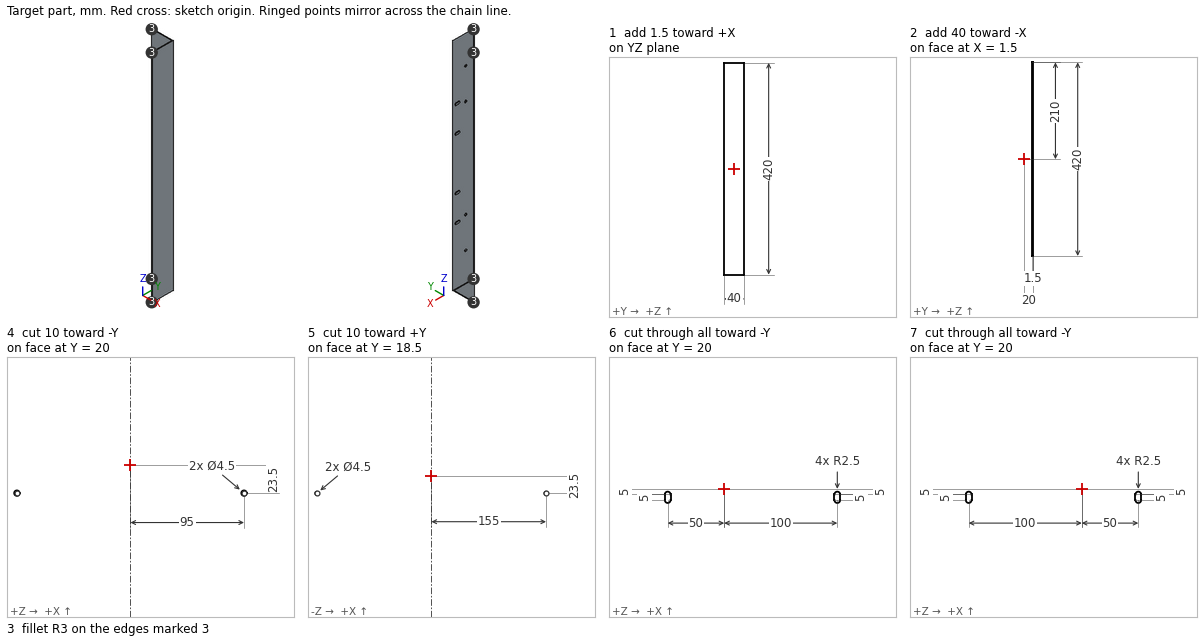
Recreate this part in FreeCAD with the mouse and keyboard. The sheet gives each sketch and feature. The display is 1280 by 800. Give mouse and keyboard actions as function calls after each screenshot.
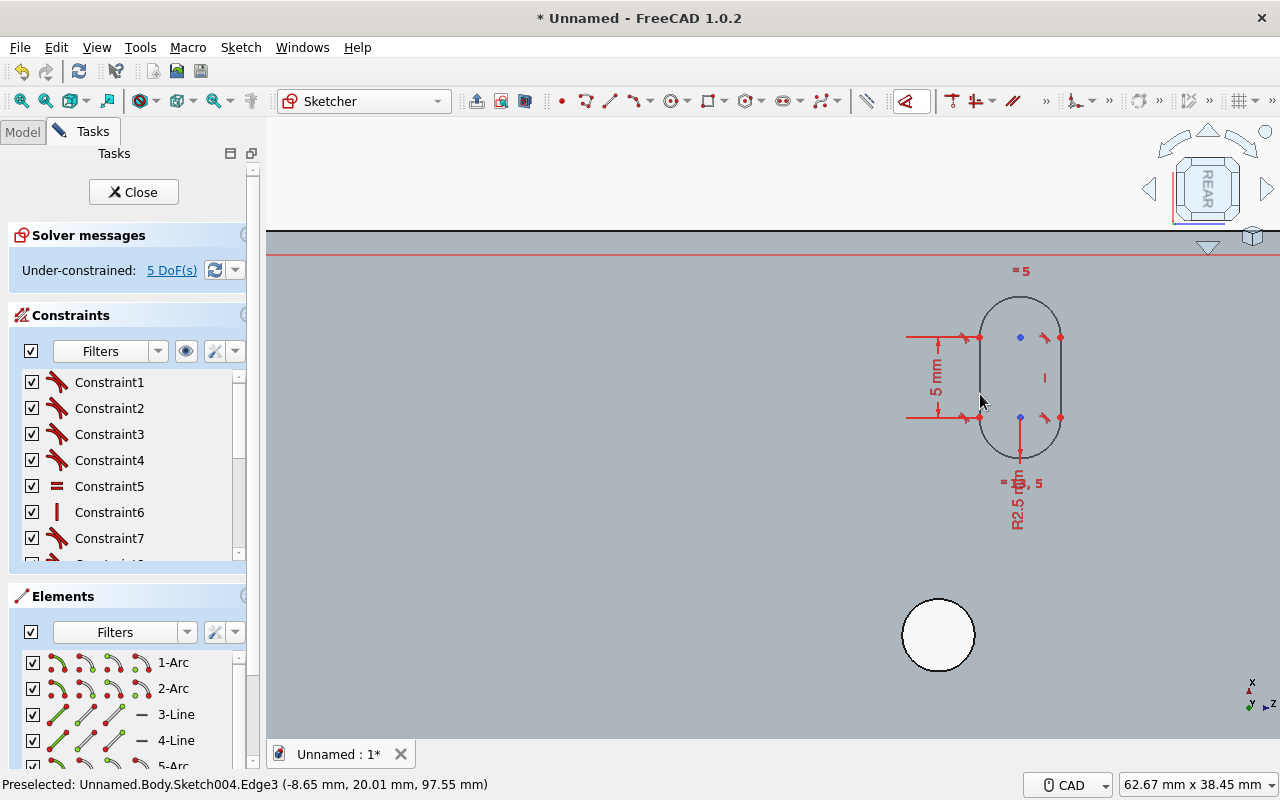
scroll(999, 452, down, 7)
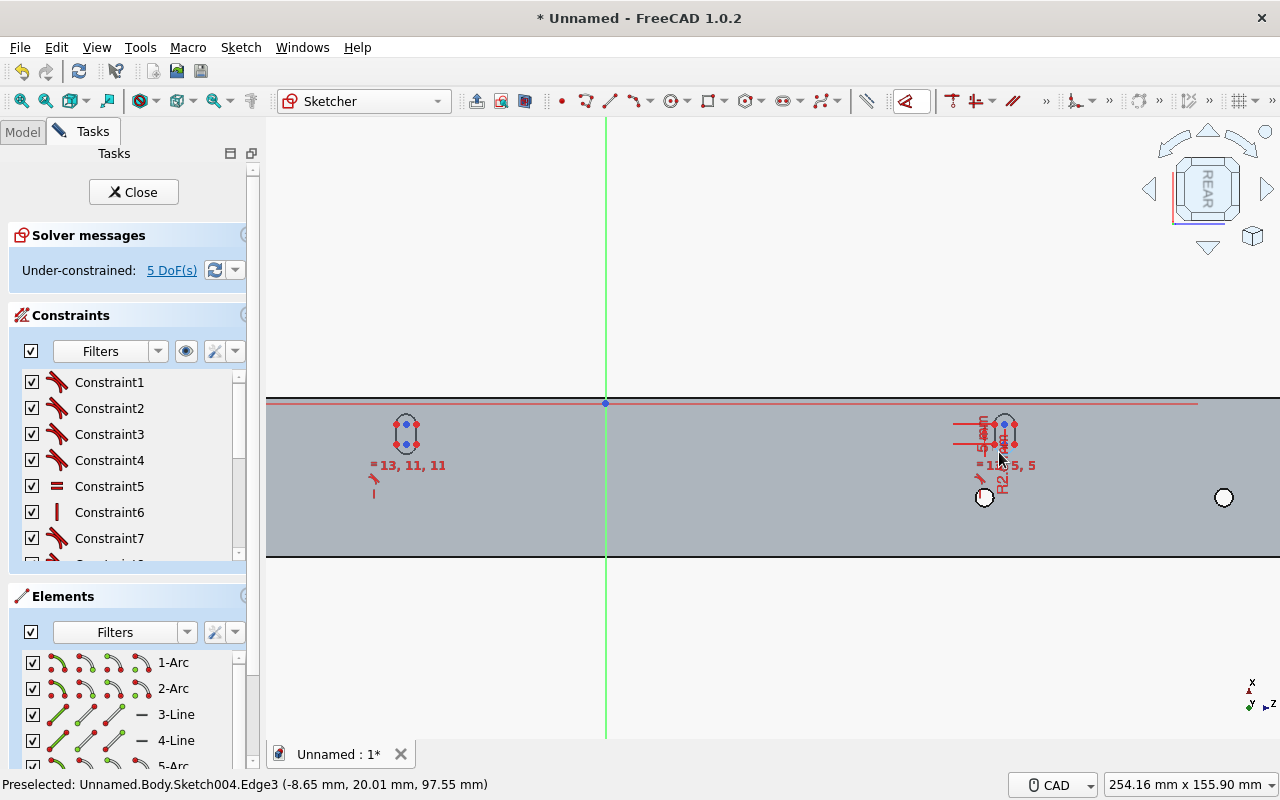
scroll(396, 438, up, 5)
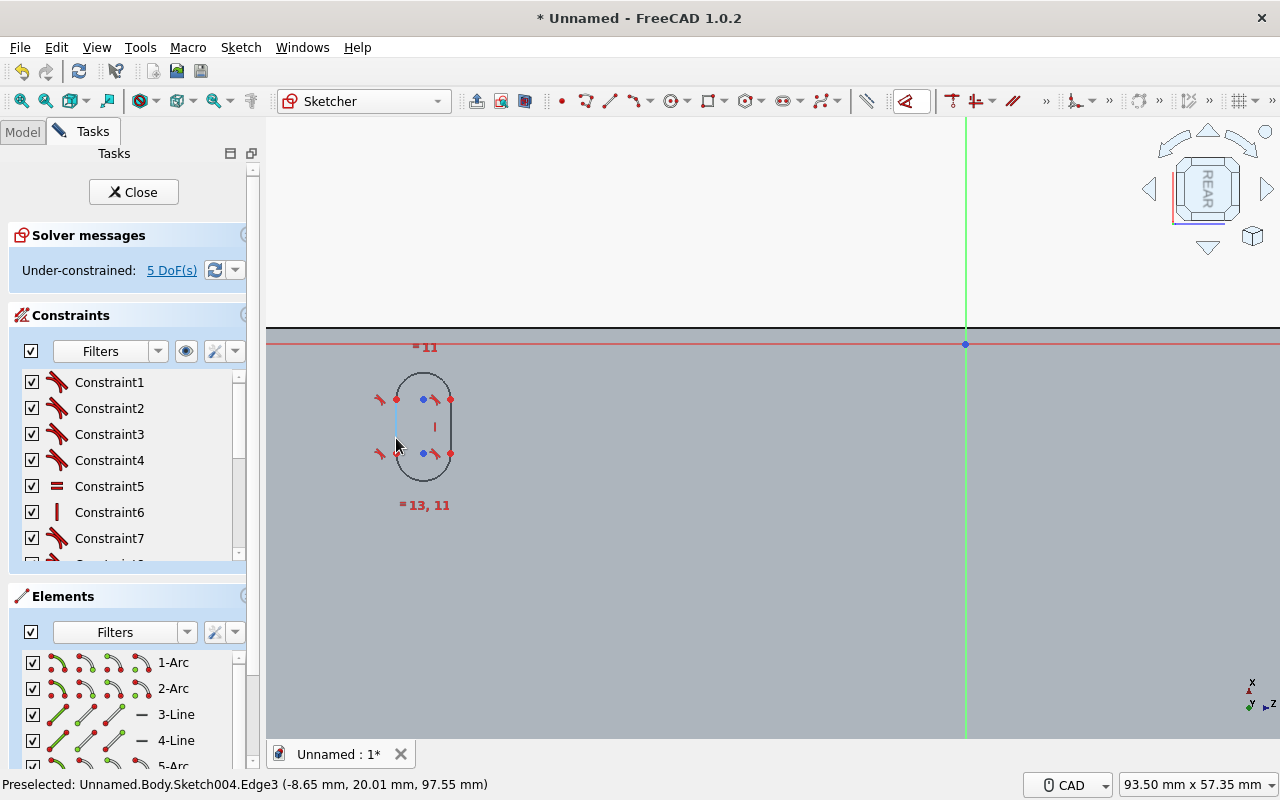
click(396, 438)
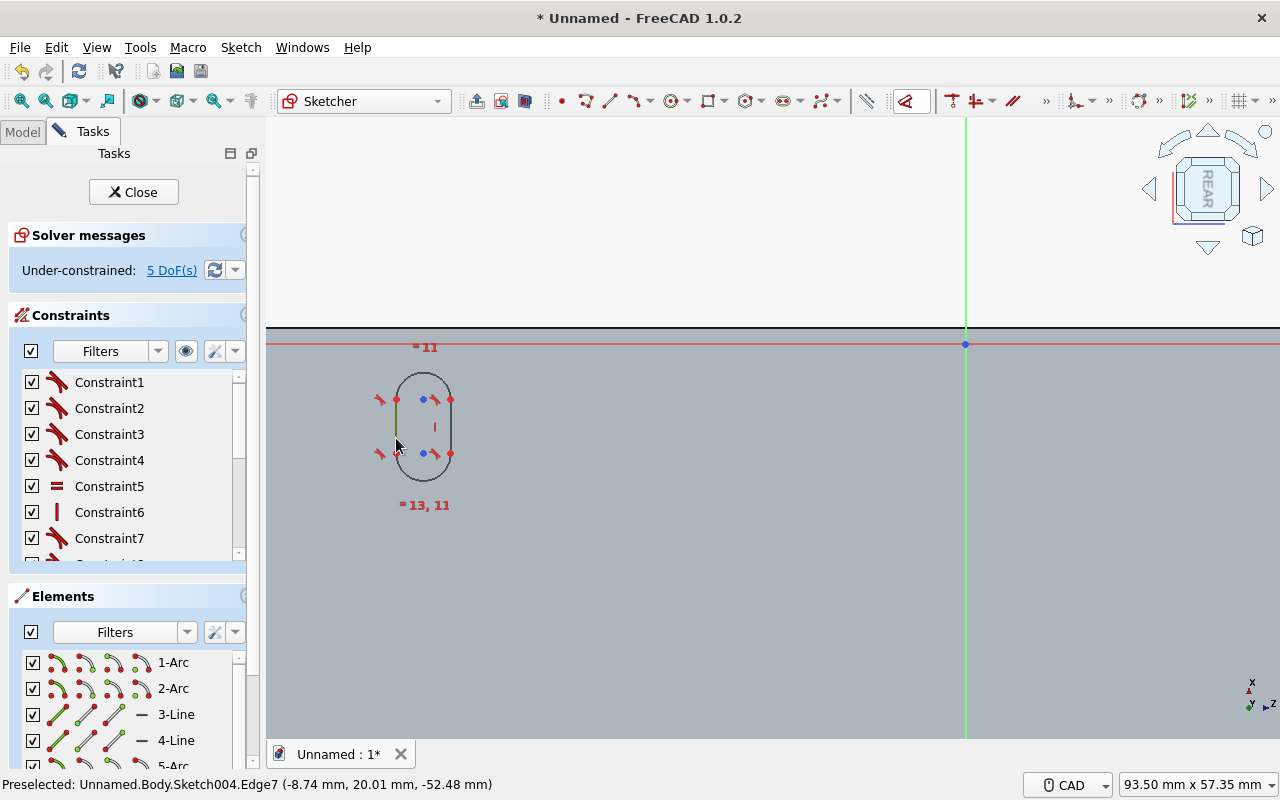
key(i)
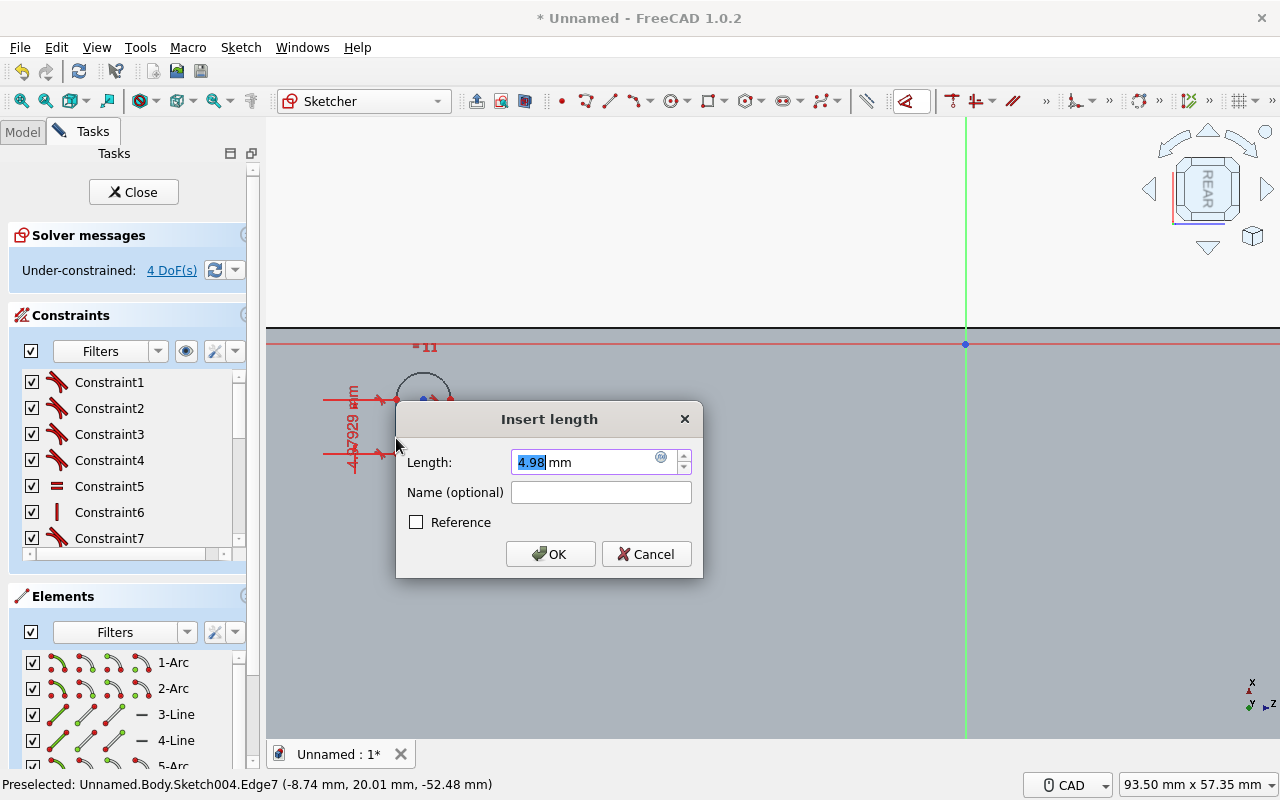
text(5)
key(Return)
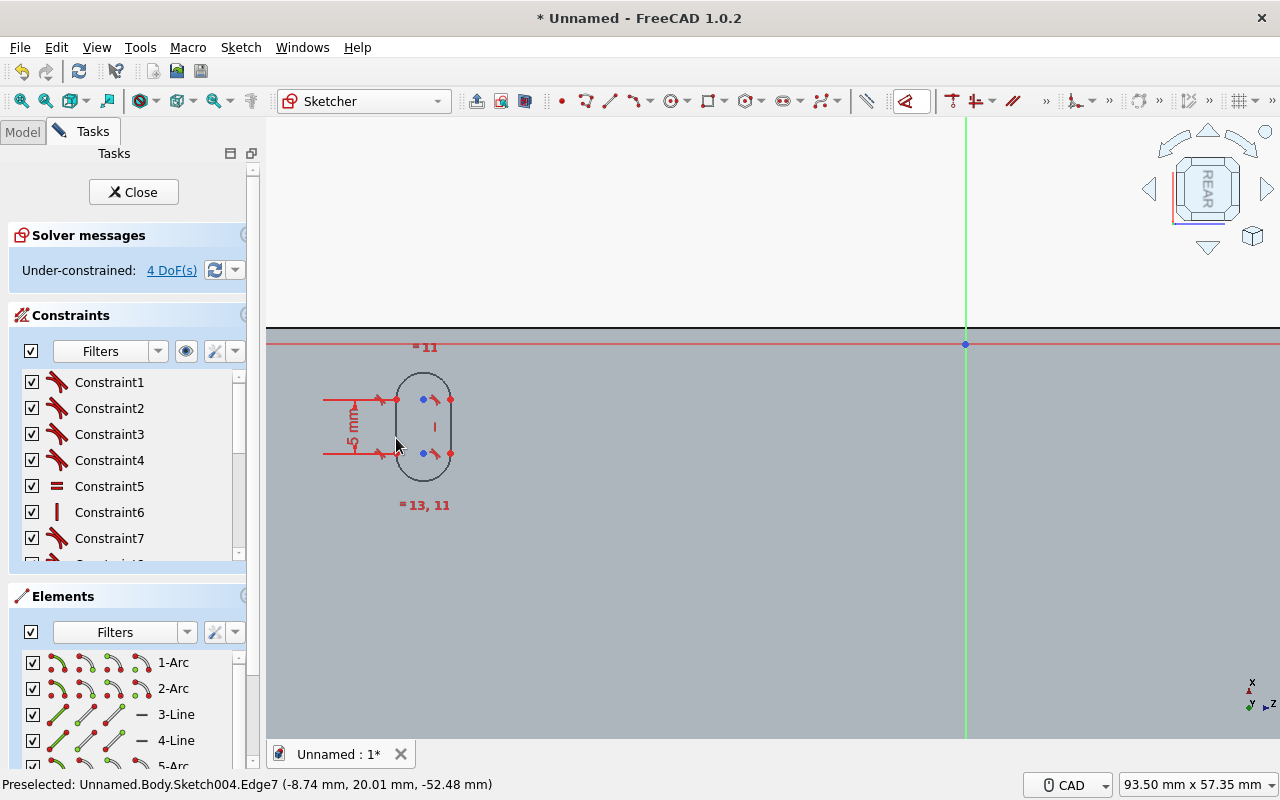
scroll(395, 437, down, 5)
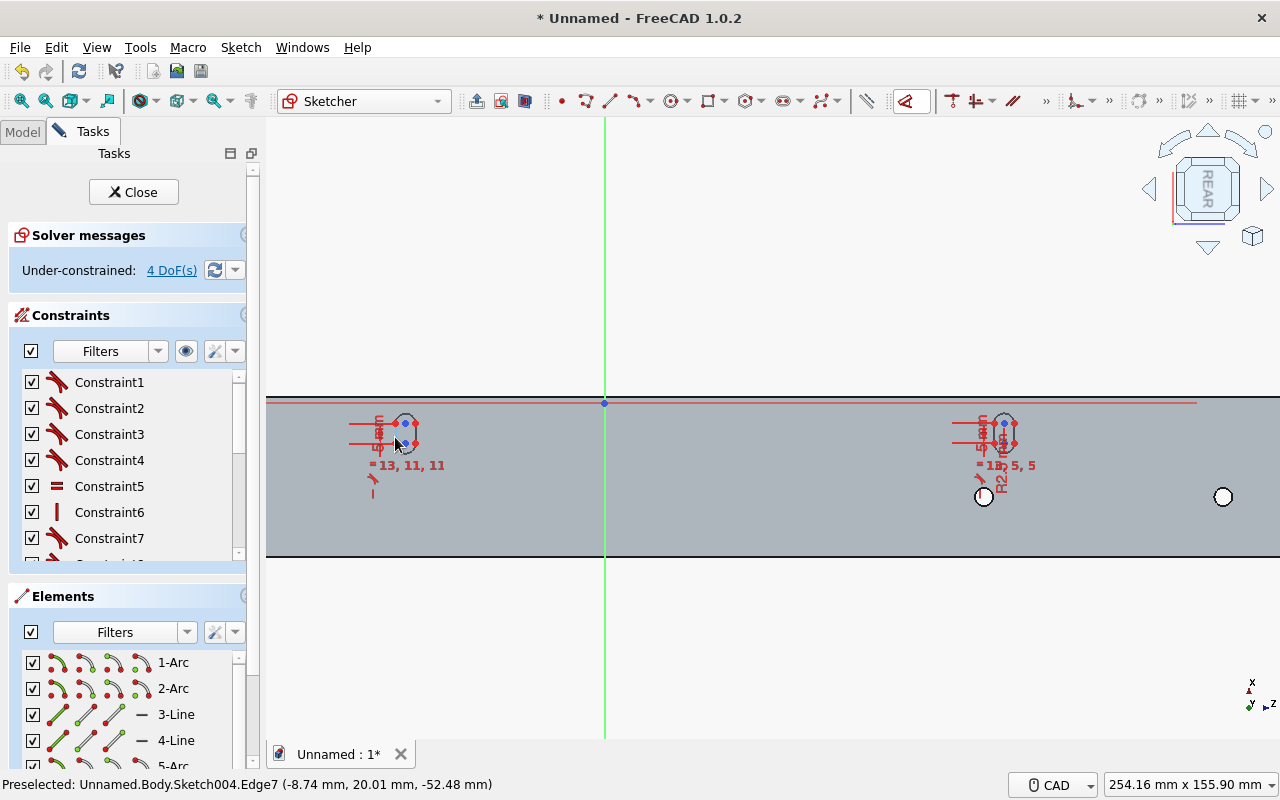
scroll(1014, 423, up, 4)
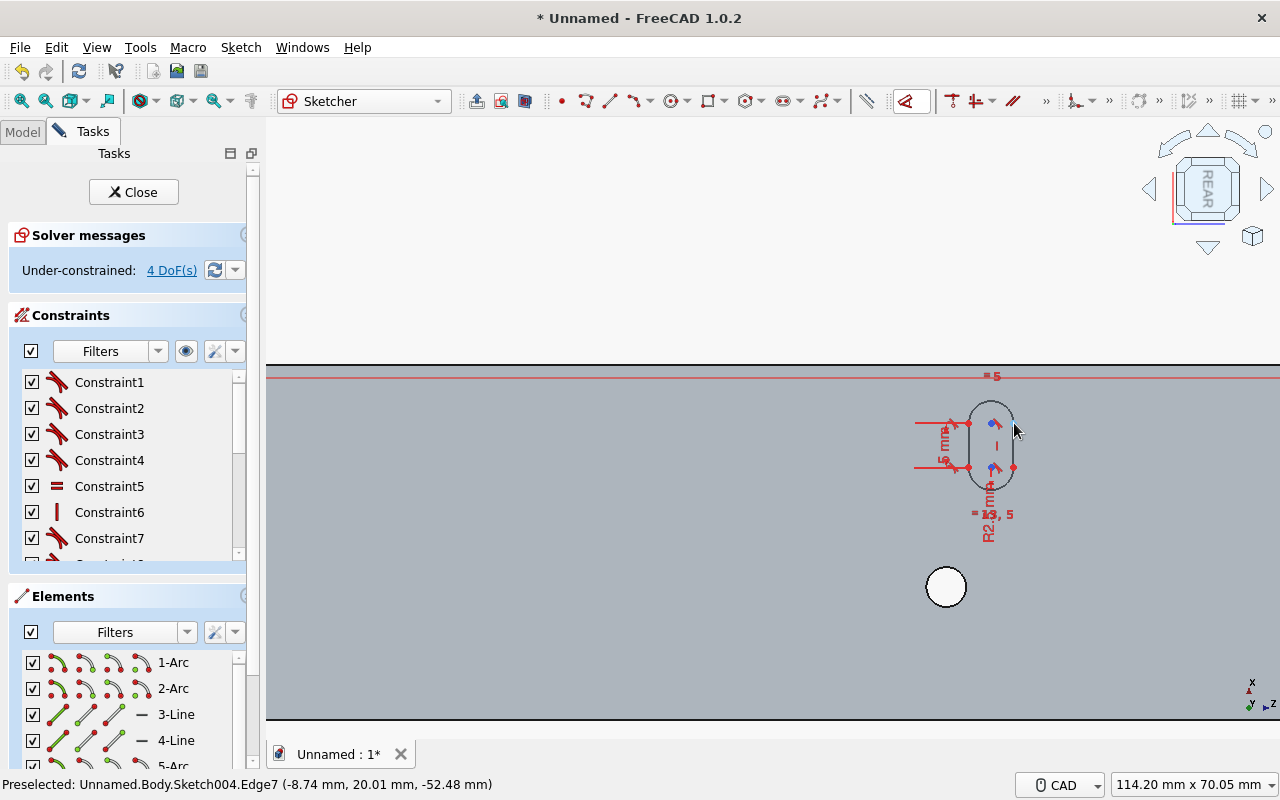
click(1013, 423)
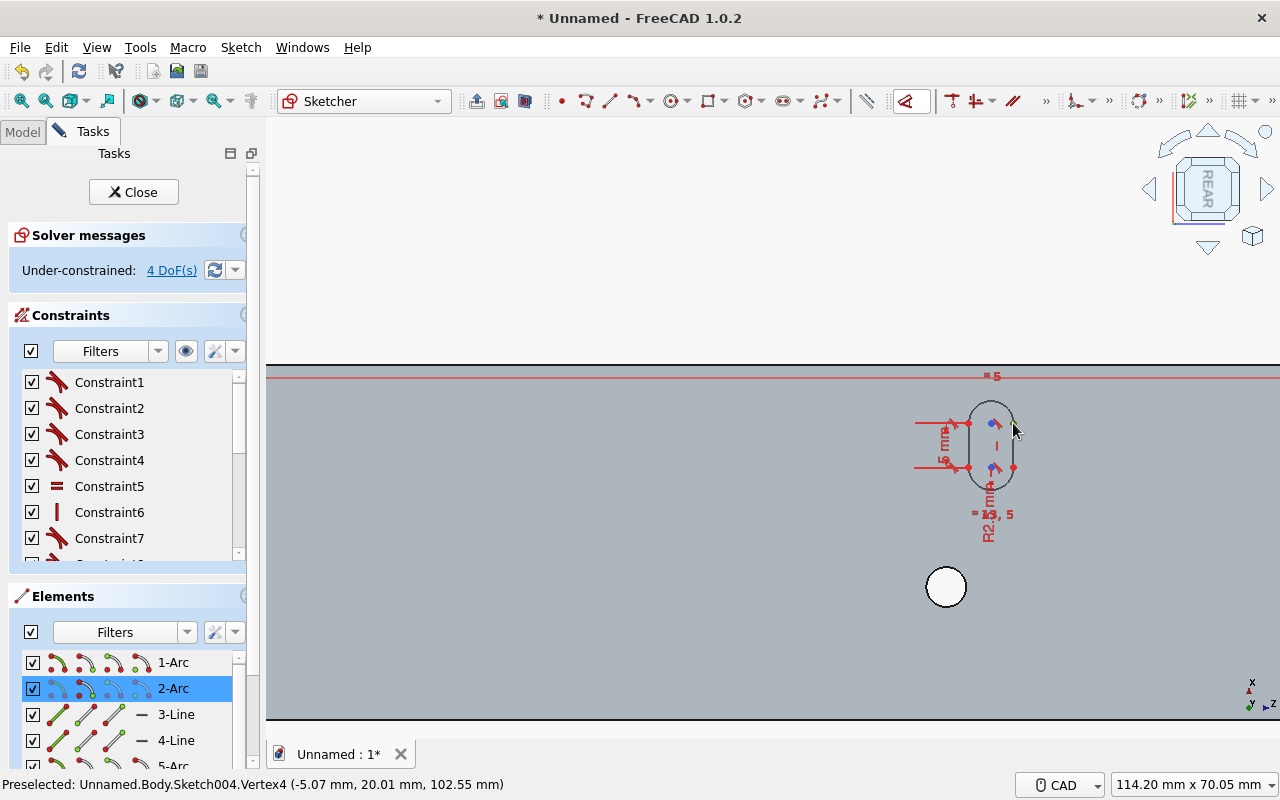
click(924, 102)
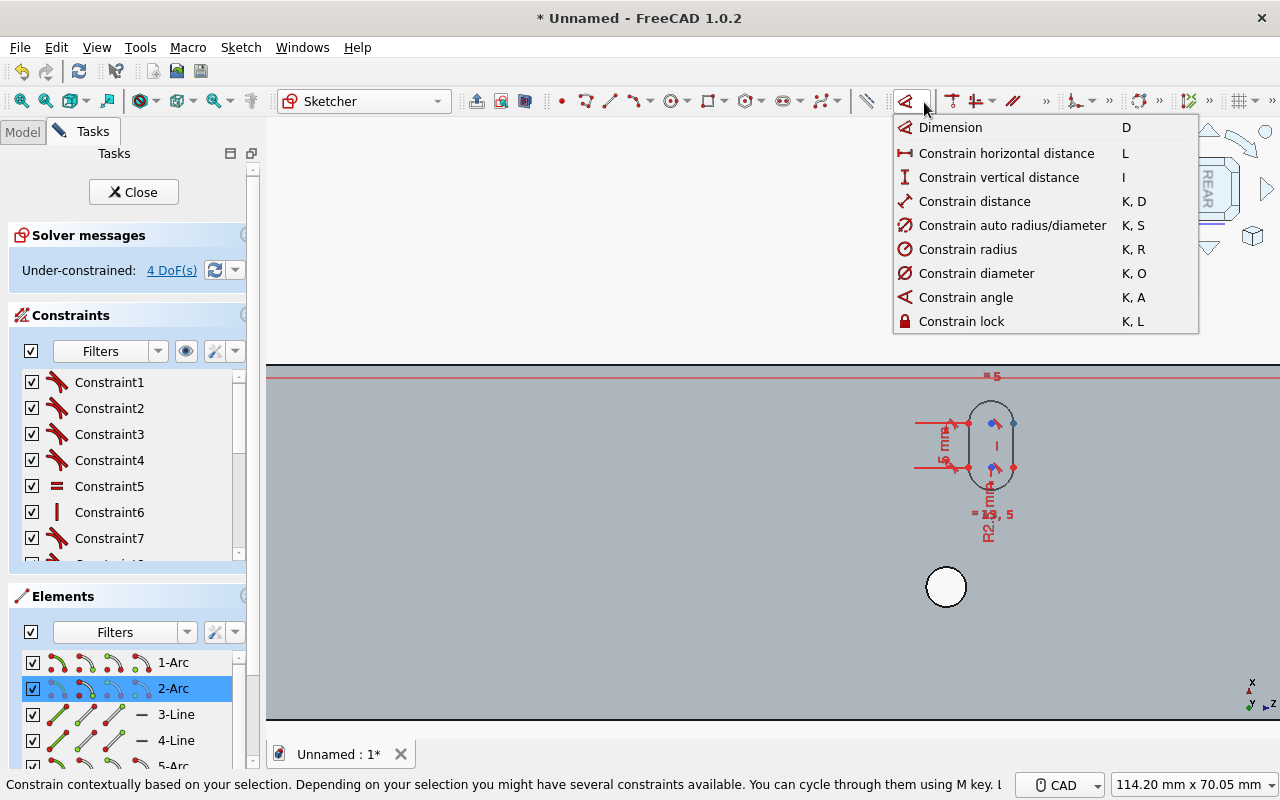
click(1046, 177)